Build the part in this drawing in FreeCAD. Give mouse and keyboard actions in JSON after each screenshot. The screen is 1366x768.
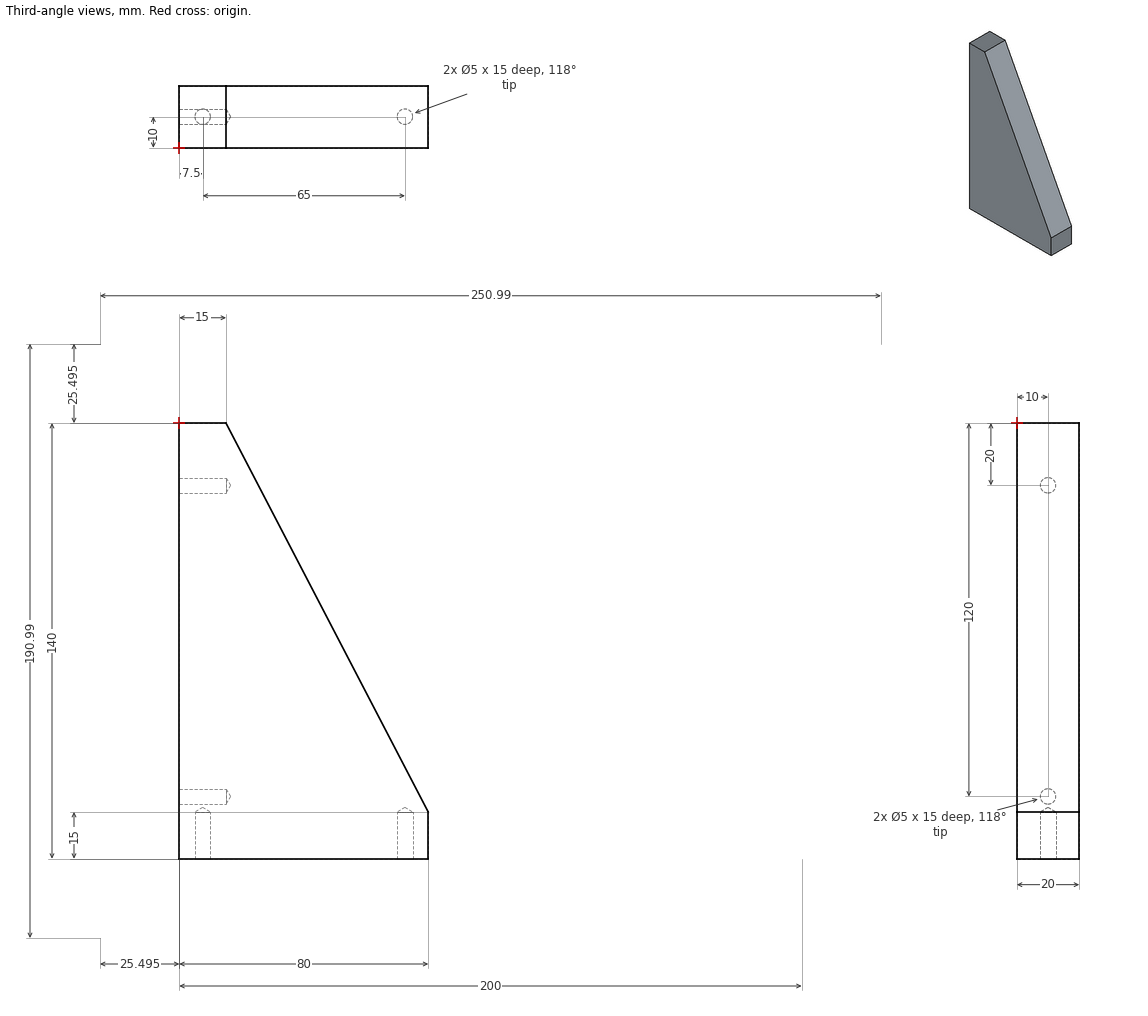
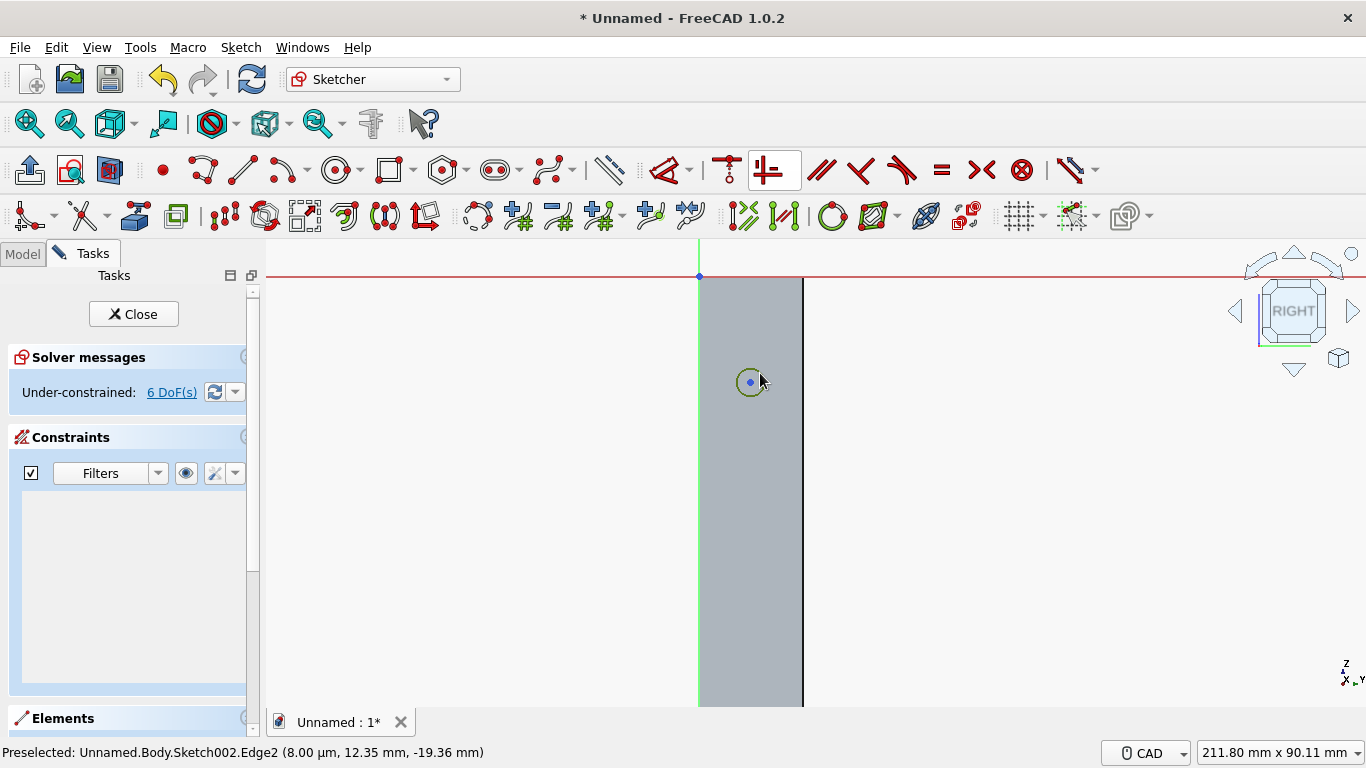
{"action": "key", "text": "e"}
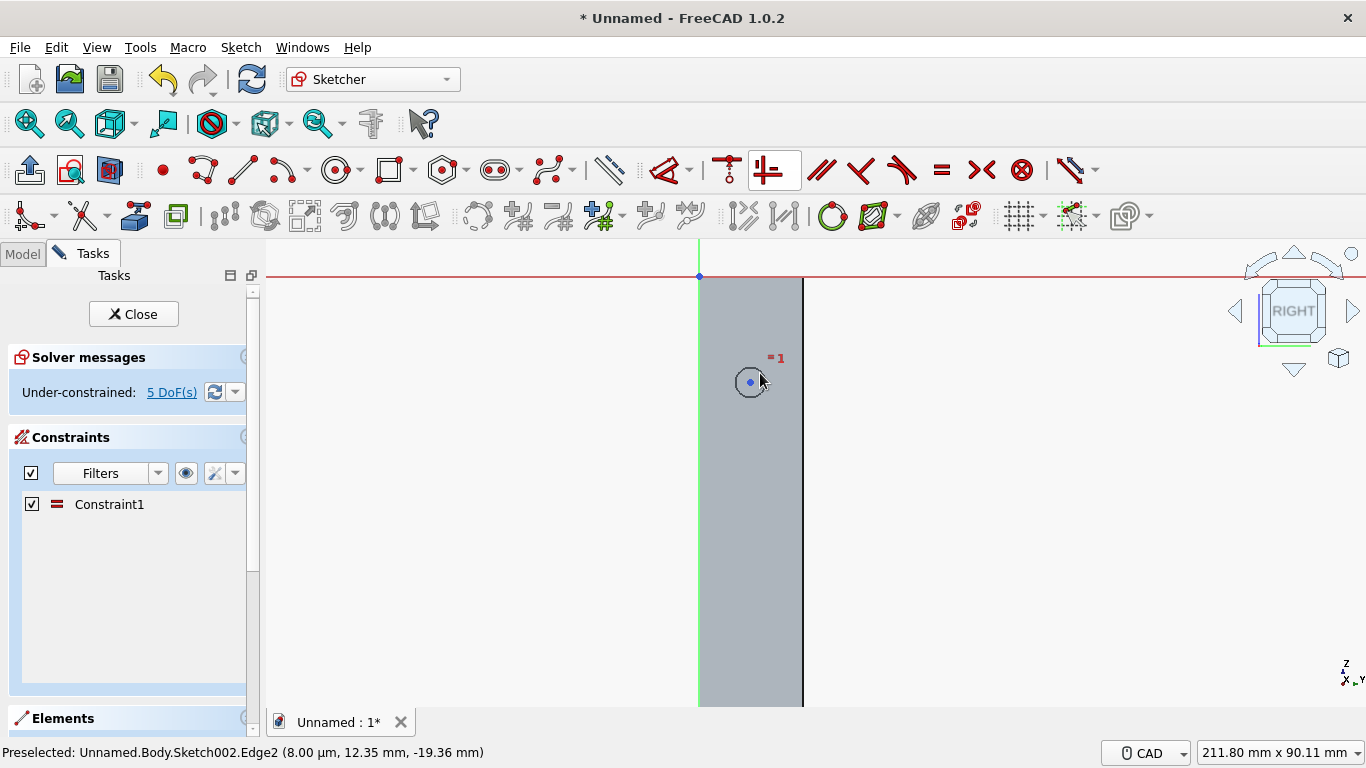
{"action": "key", "text": "d"}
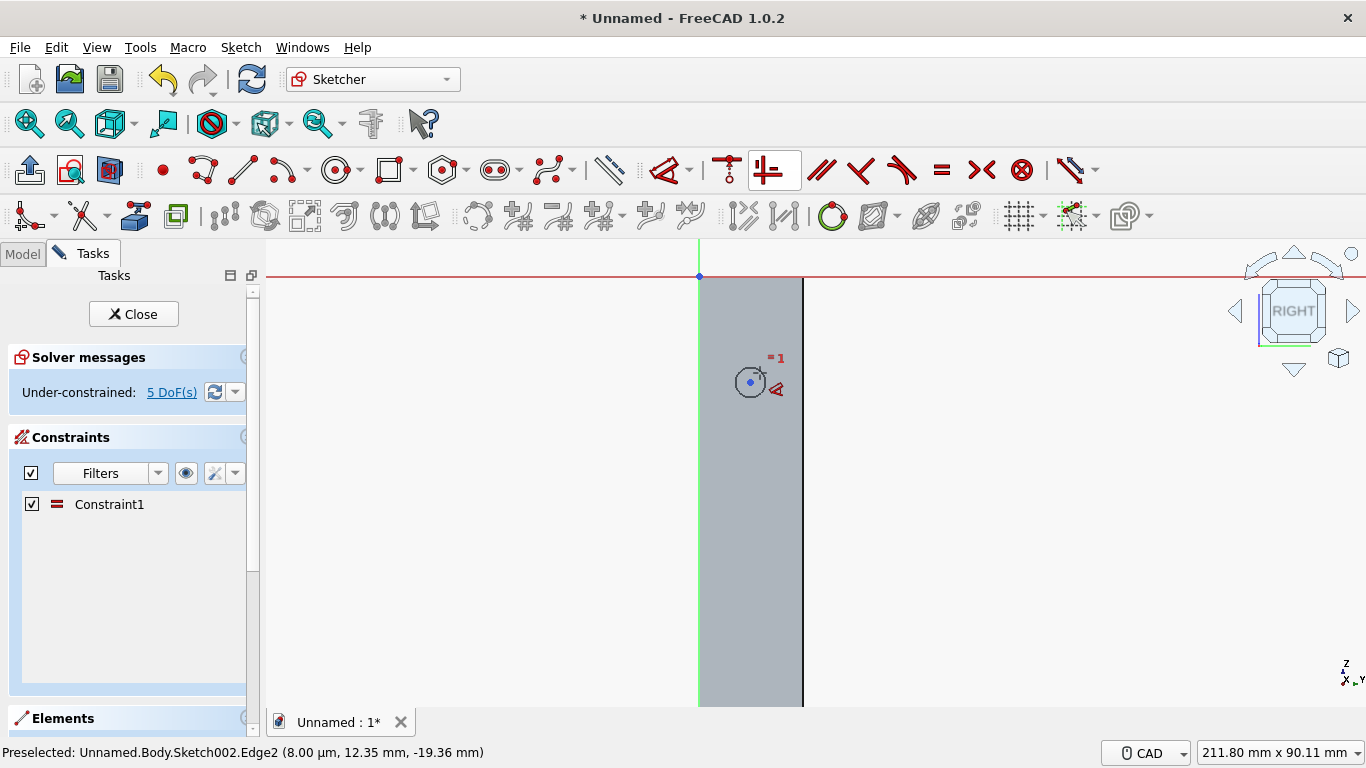
{"action": "scroll", "coordinate": [760, 373], "scroll_direction": "down", "scroll_amount": 4}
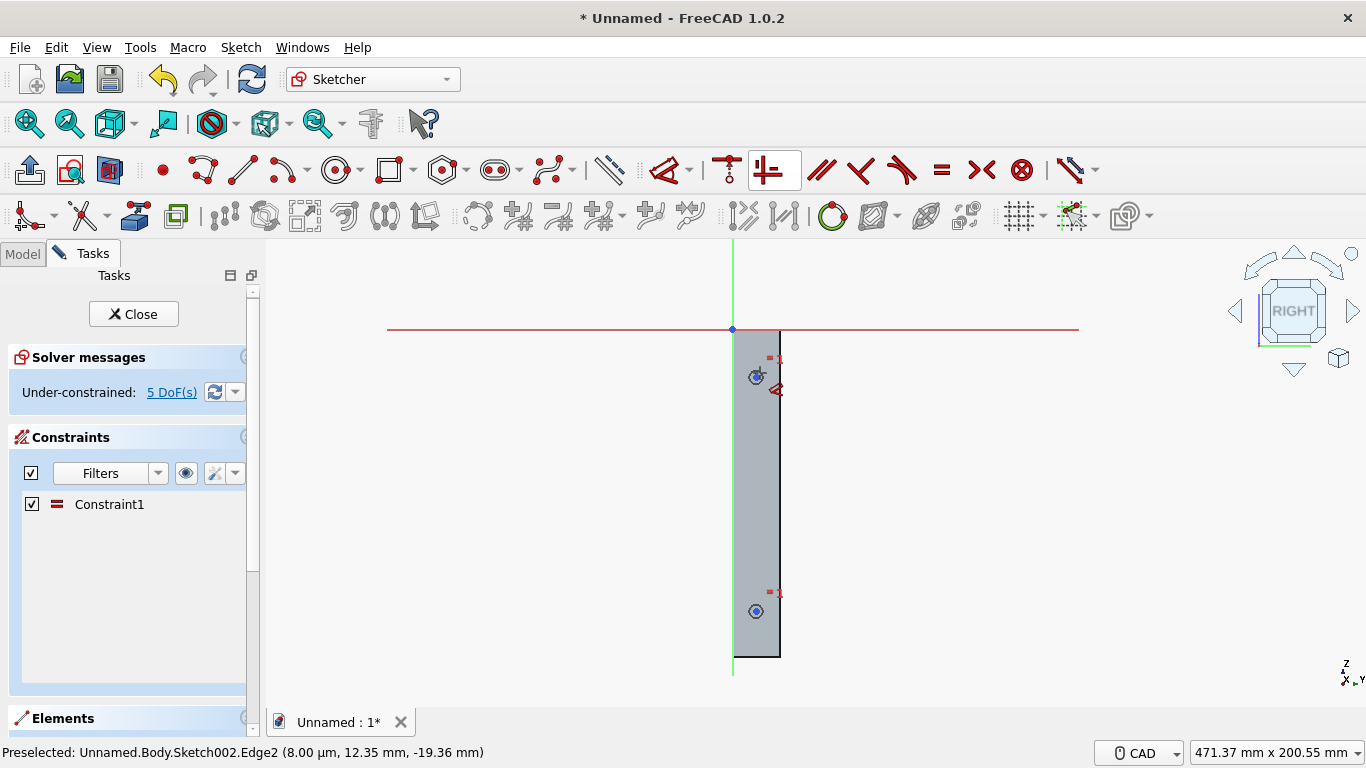
{"action": "scroll", "coordinate": [761, 607], "scroll_direction": "up", "scroll_amount": 7}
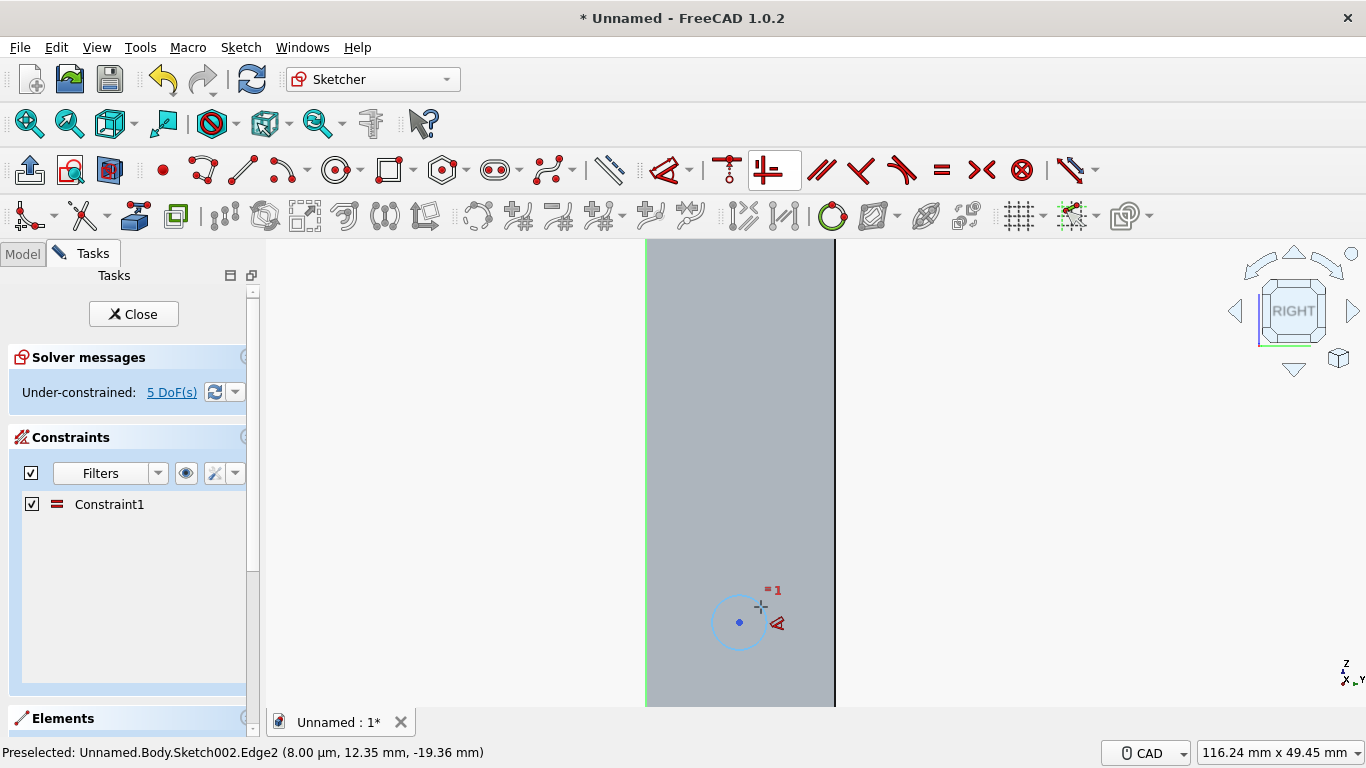
{"action": "left_click", "coordinate": [759, 603]}
{"action": "left_click", "coordinate": [782, 580]}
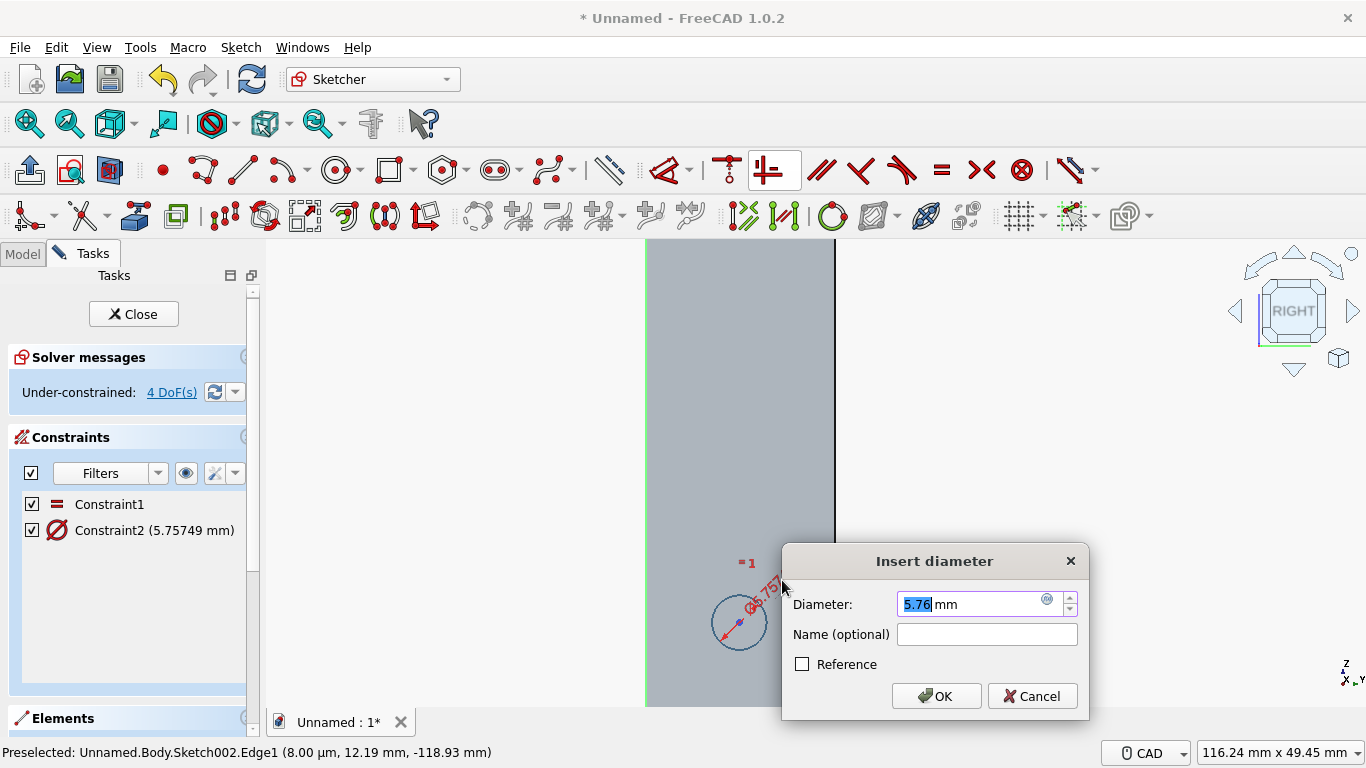
{"action": "type", "text": "5"}
{"action": "key", "text": "Return"}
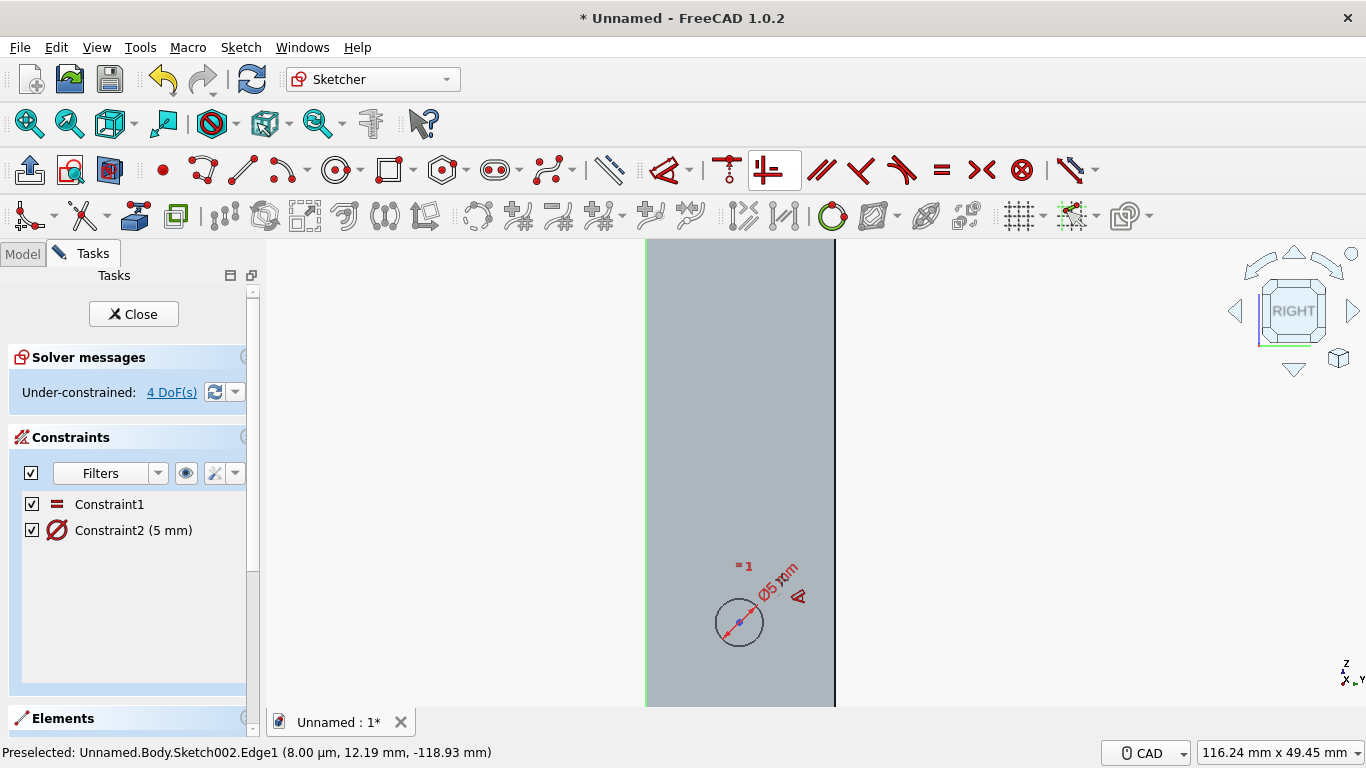
{"action": "left_click", "coordinate": [739, 623]}
{"action": "left_click", "coordinate": [693, 657]}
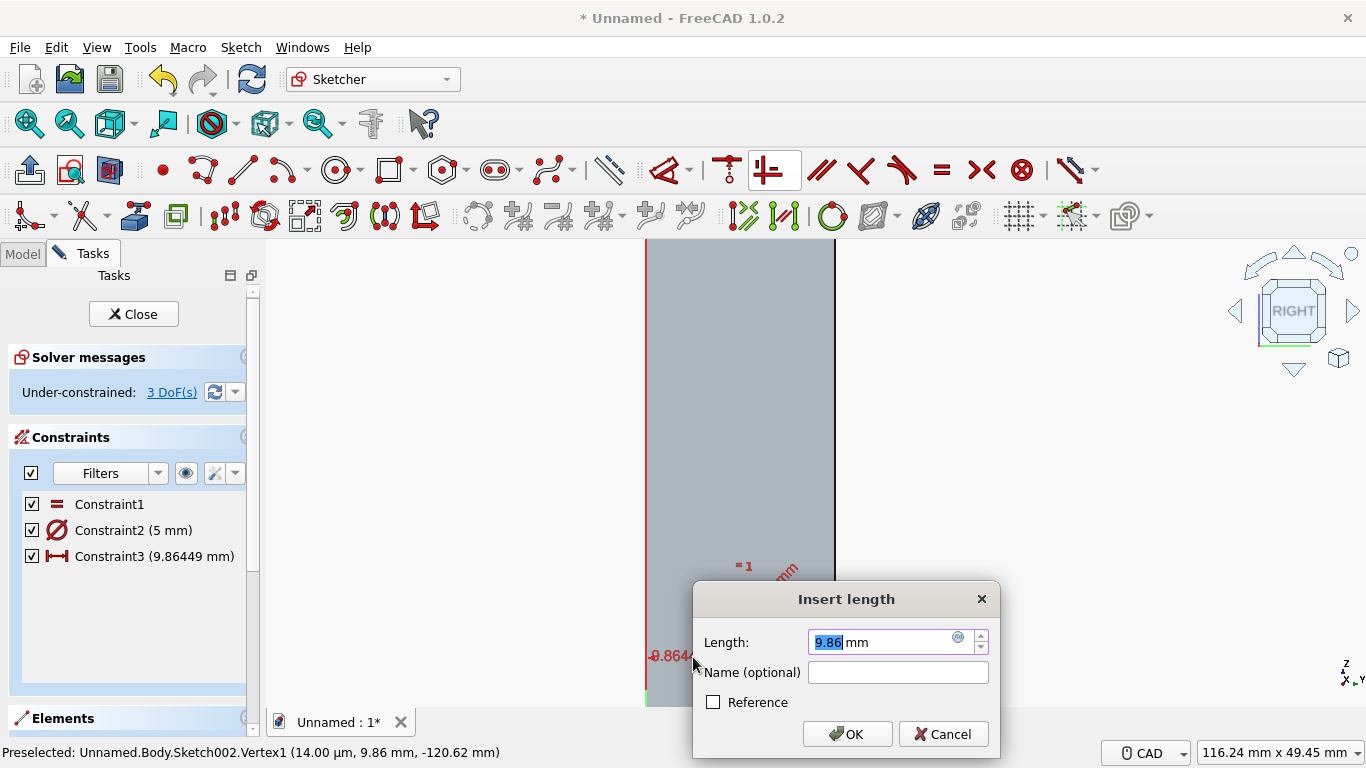
{"action": "type", "text": "10"}
{"action": "key", "text": "Return"}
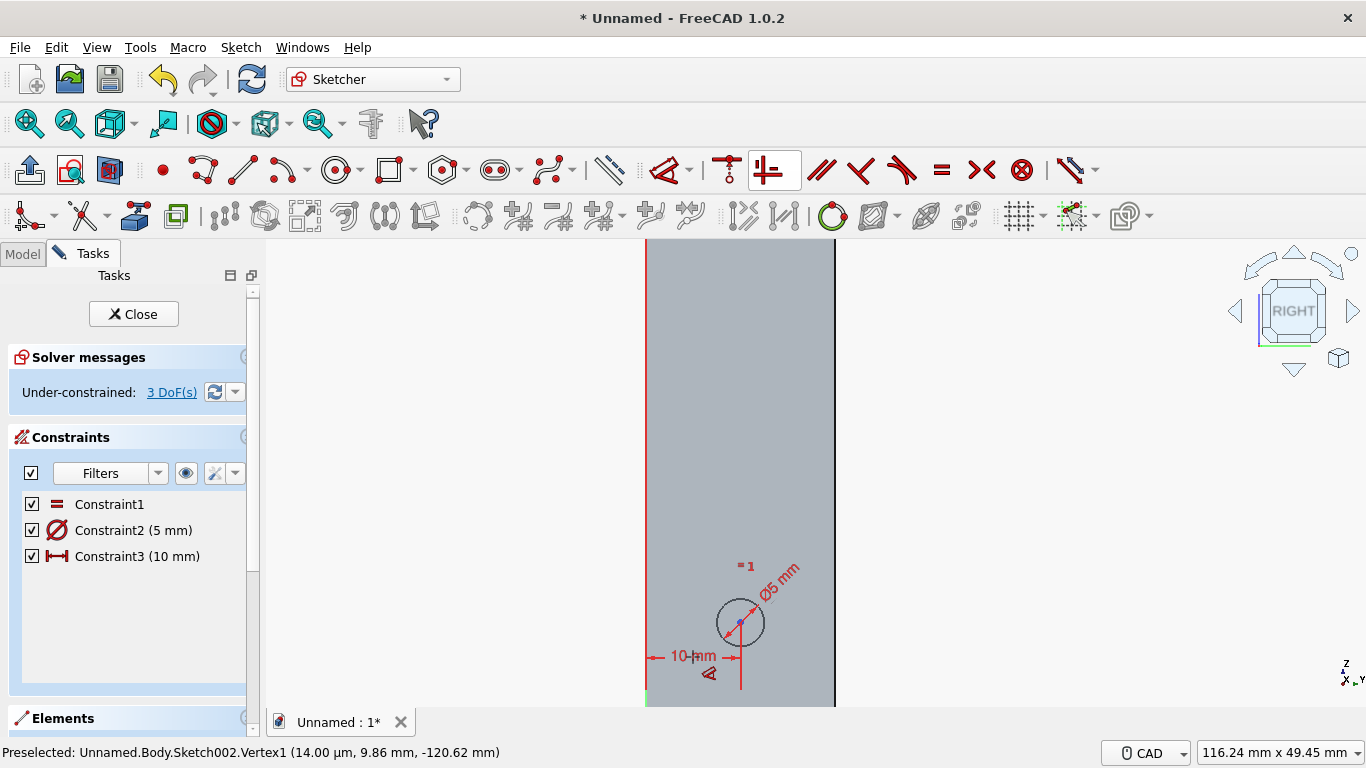
{"action": "scroll", "coordinate": [761, 608], "scroll_direction": "down", "scroll_amount": 7}